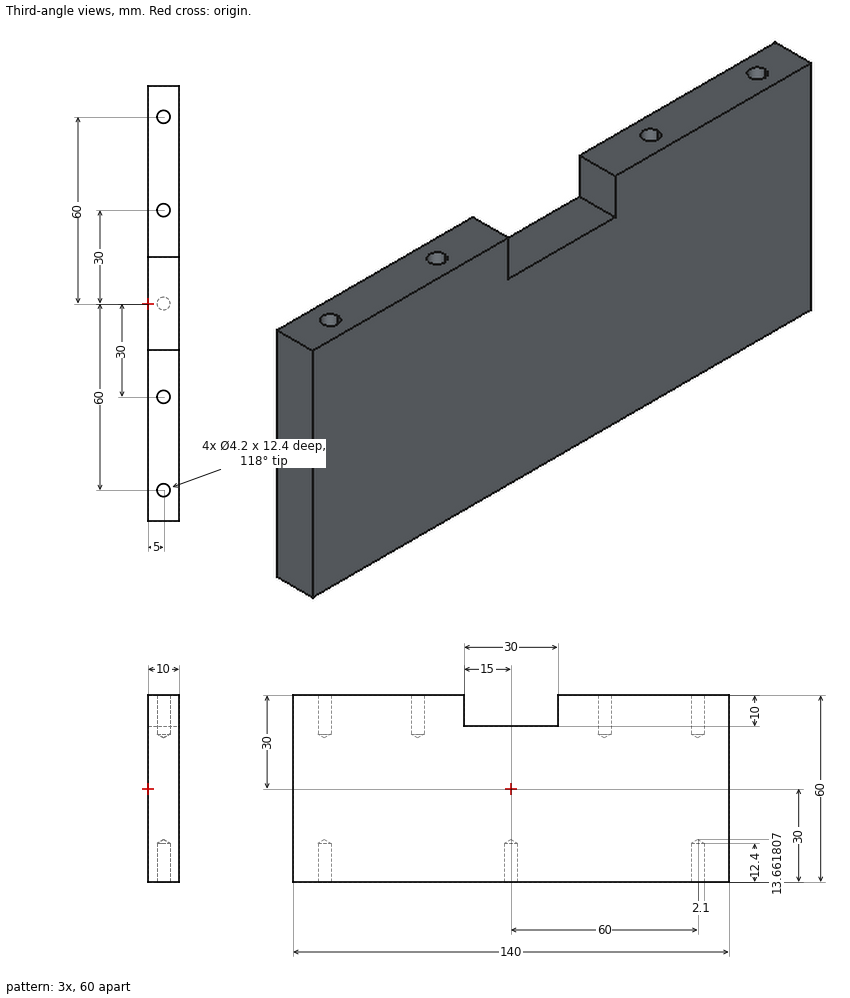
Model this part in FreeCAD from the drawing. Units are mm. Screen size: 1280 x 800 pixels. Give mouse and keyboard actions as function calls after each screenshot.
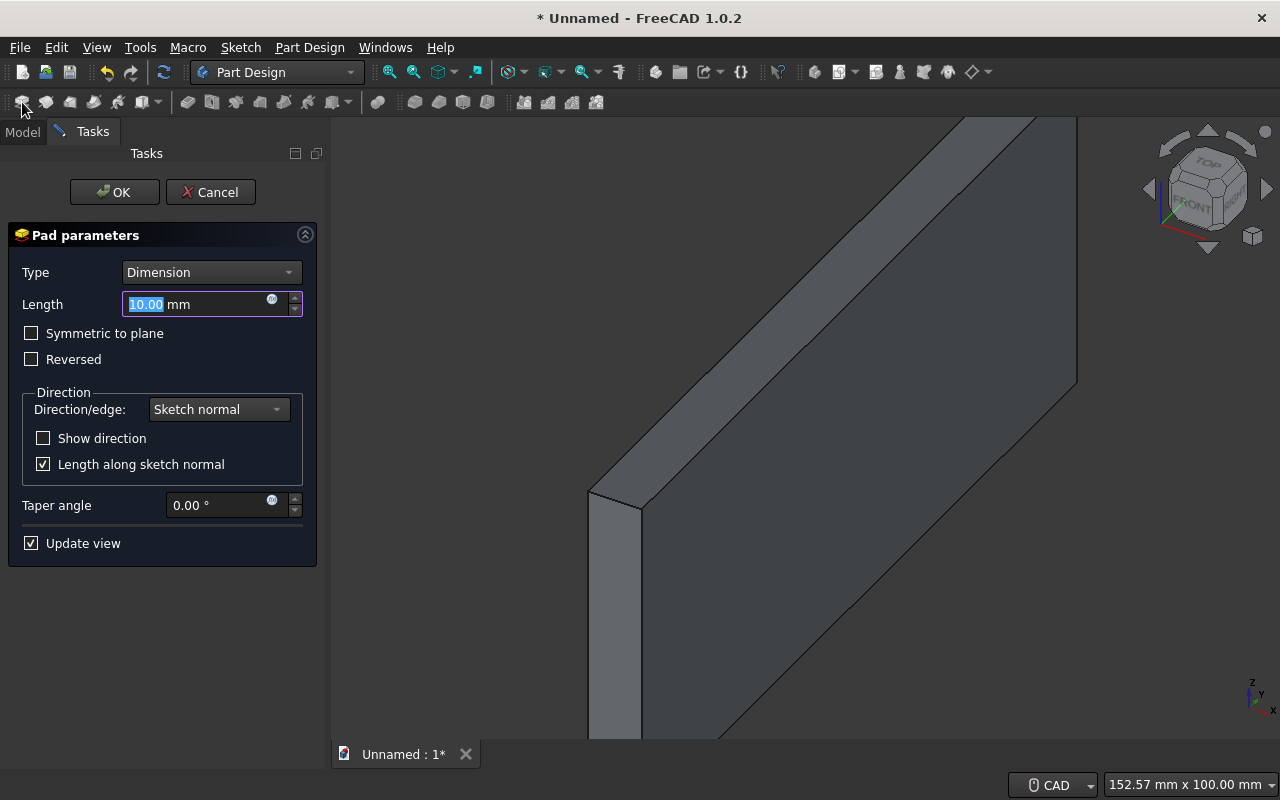
text(10)
key(Tab)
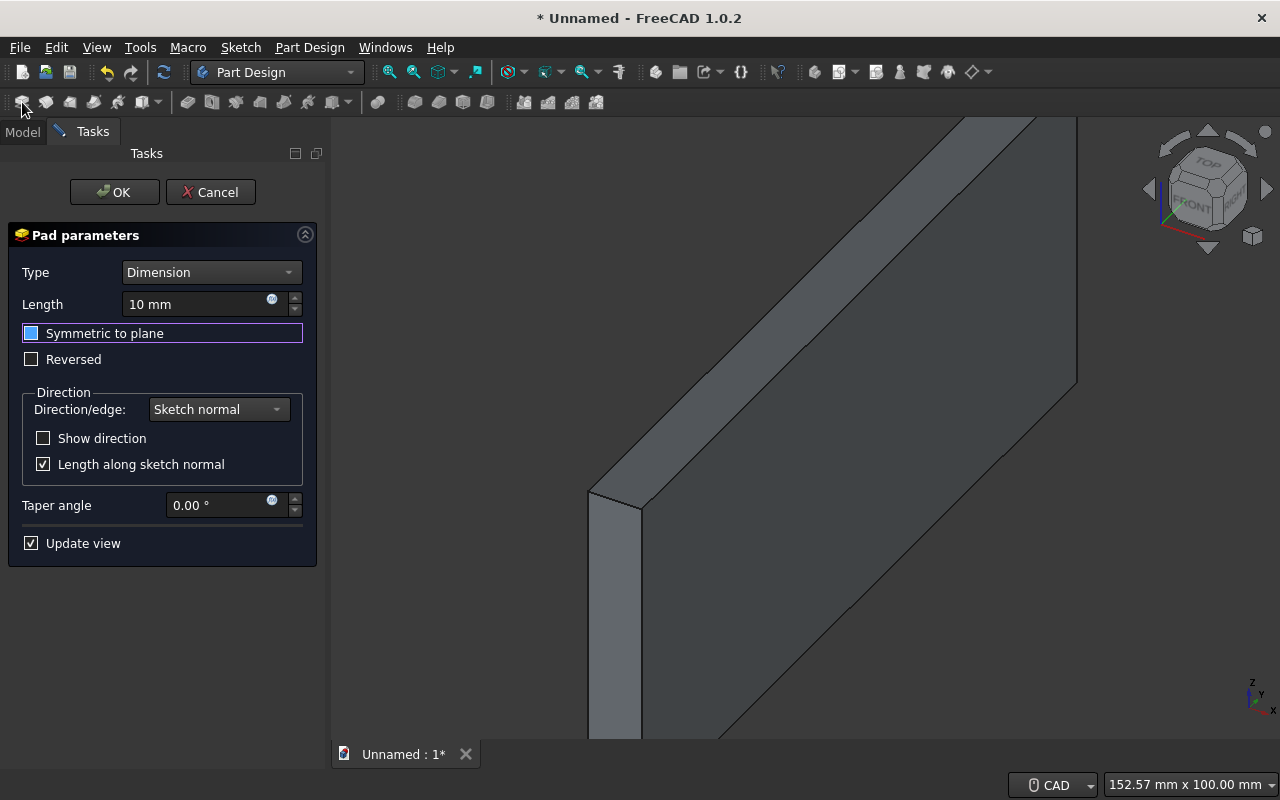
click(115, 192)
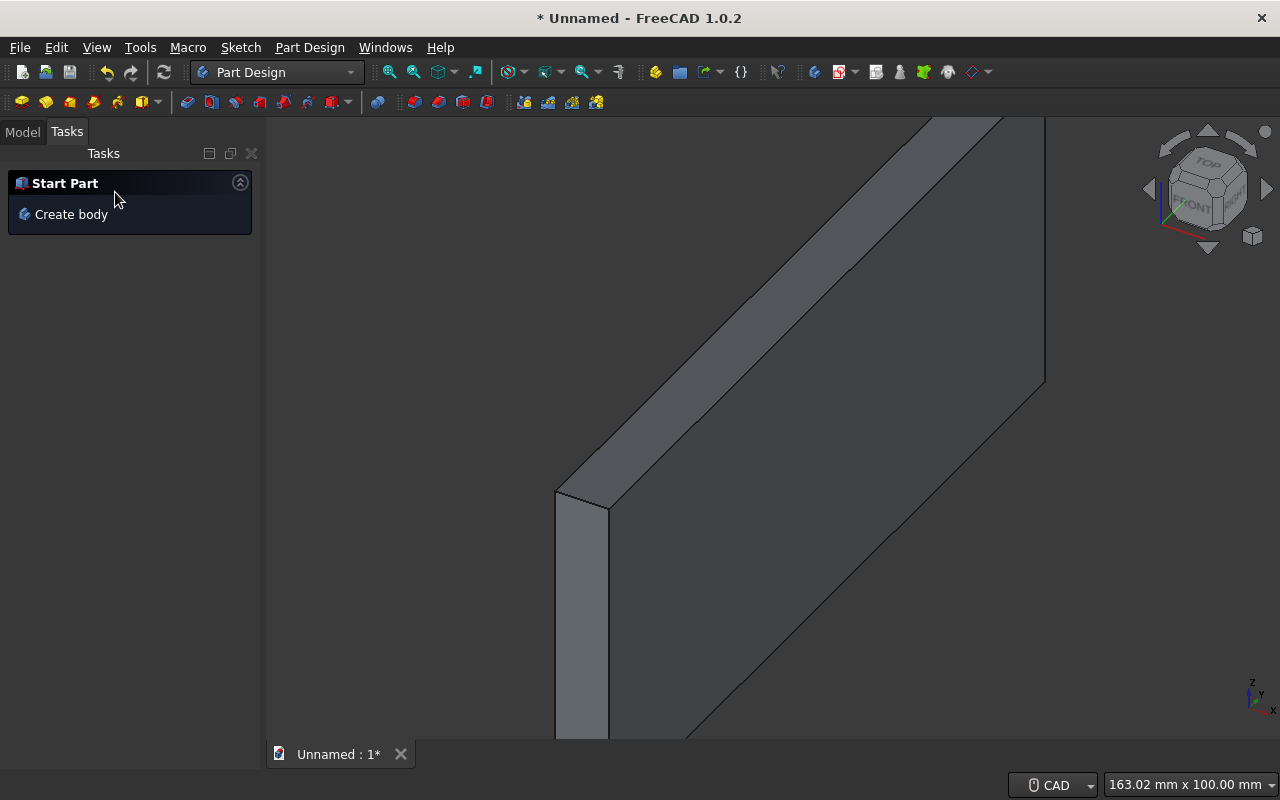
click(390, 72)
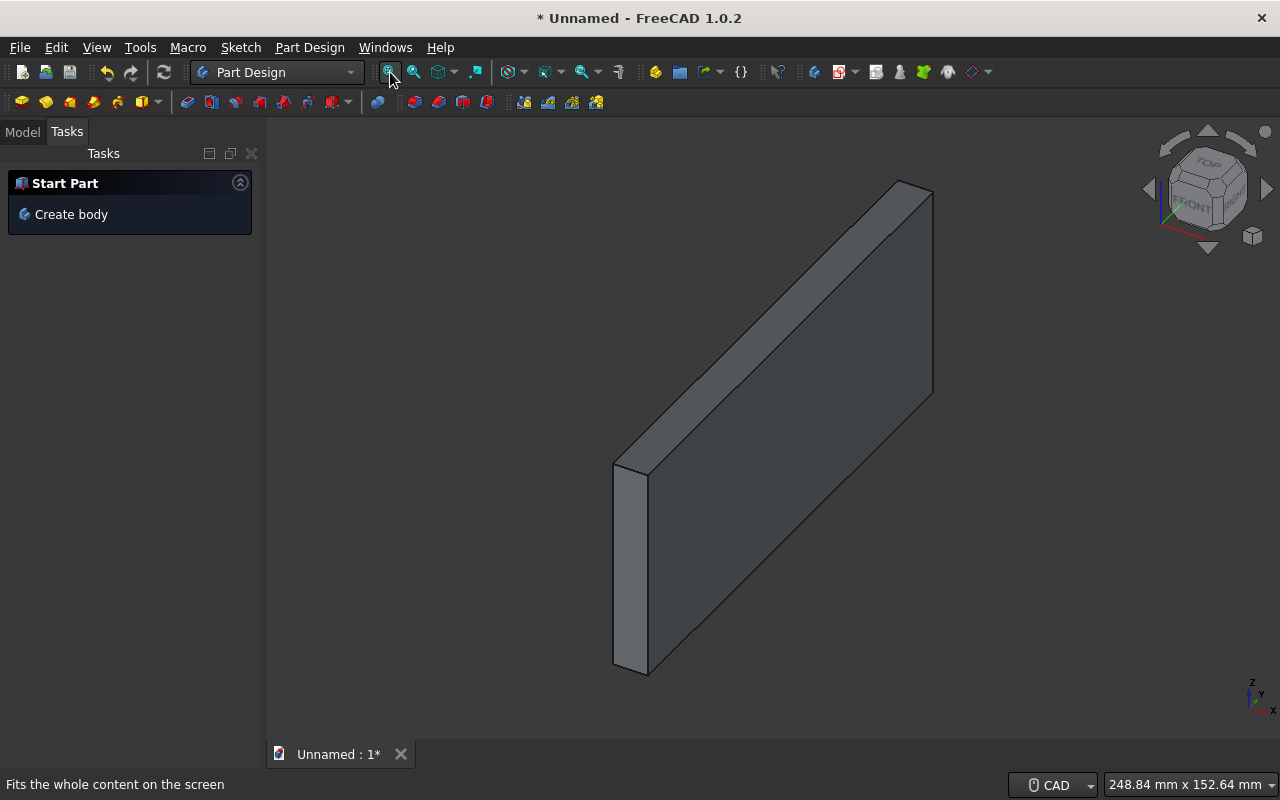
click(840, 72)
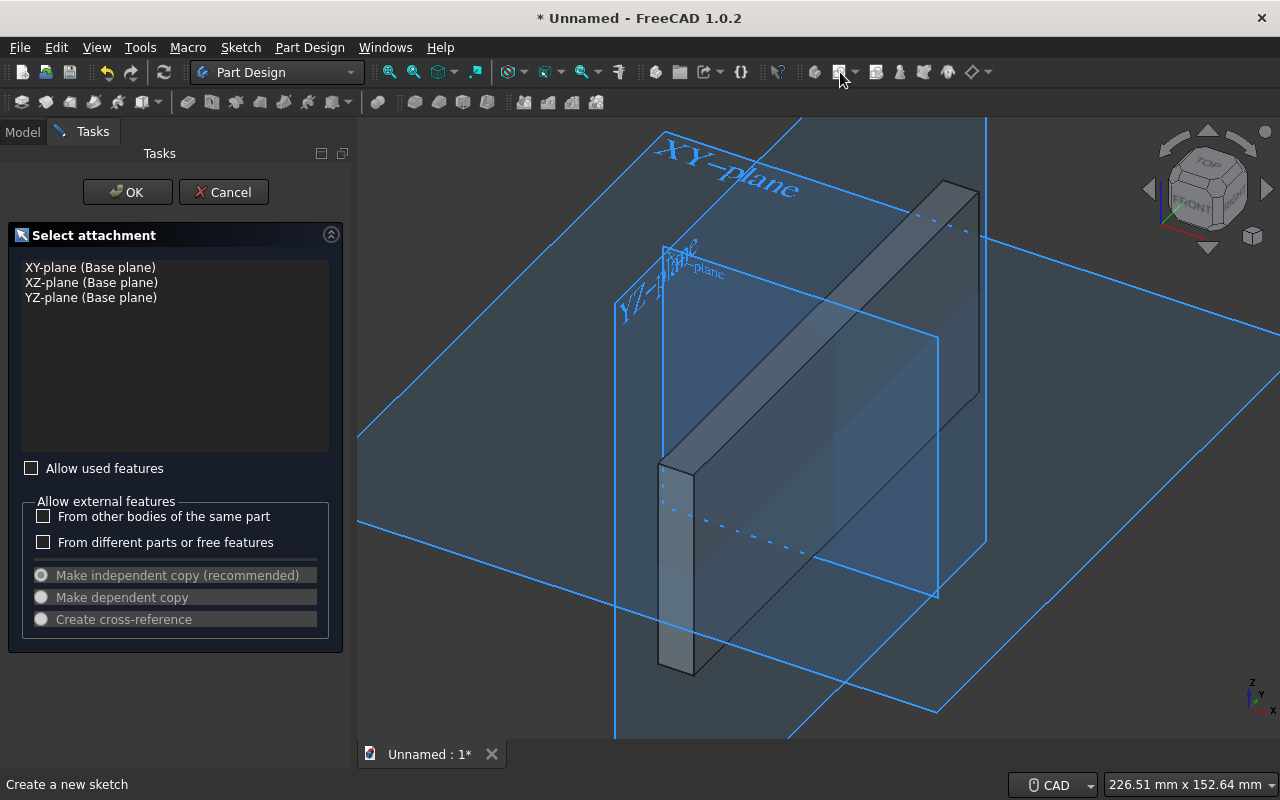
click(82, 298)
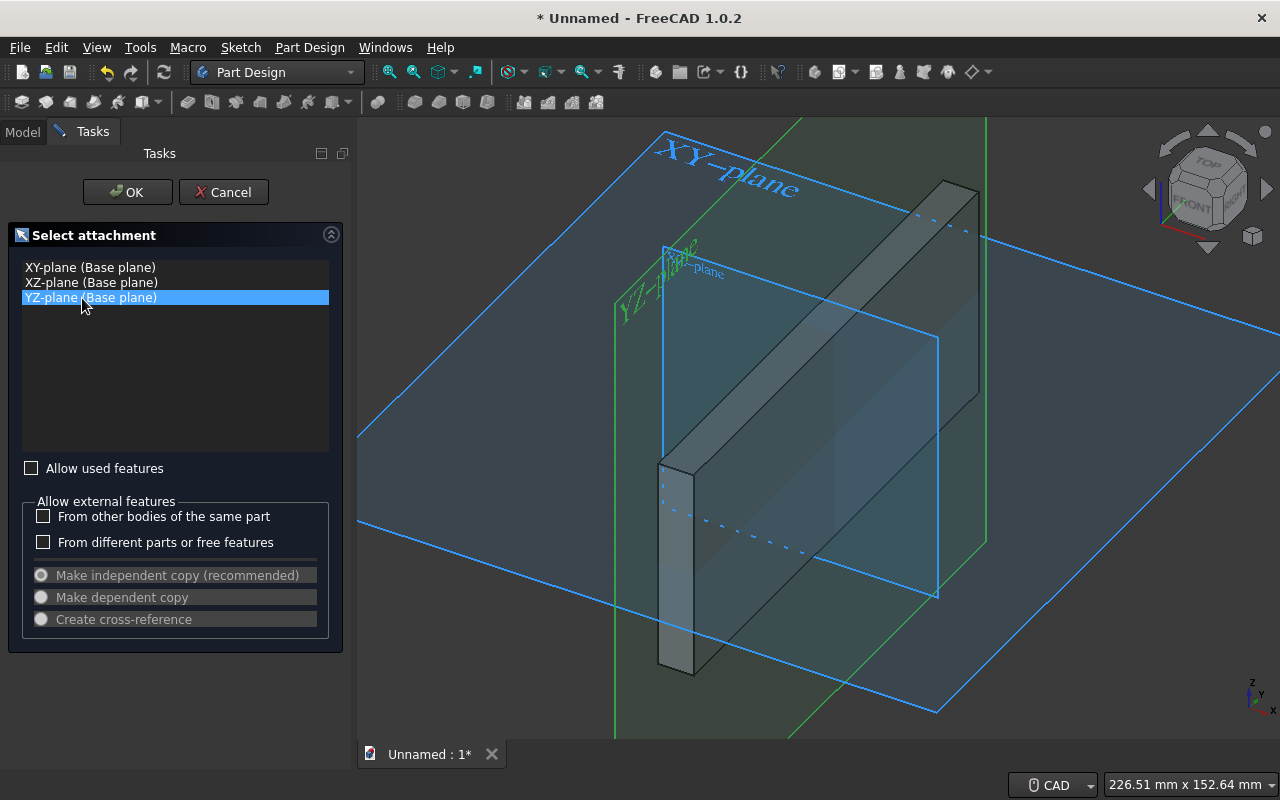
click(128, 192)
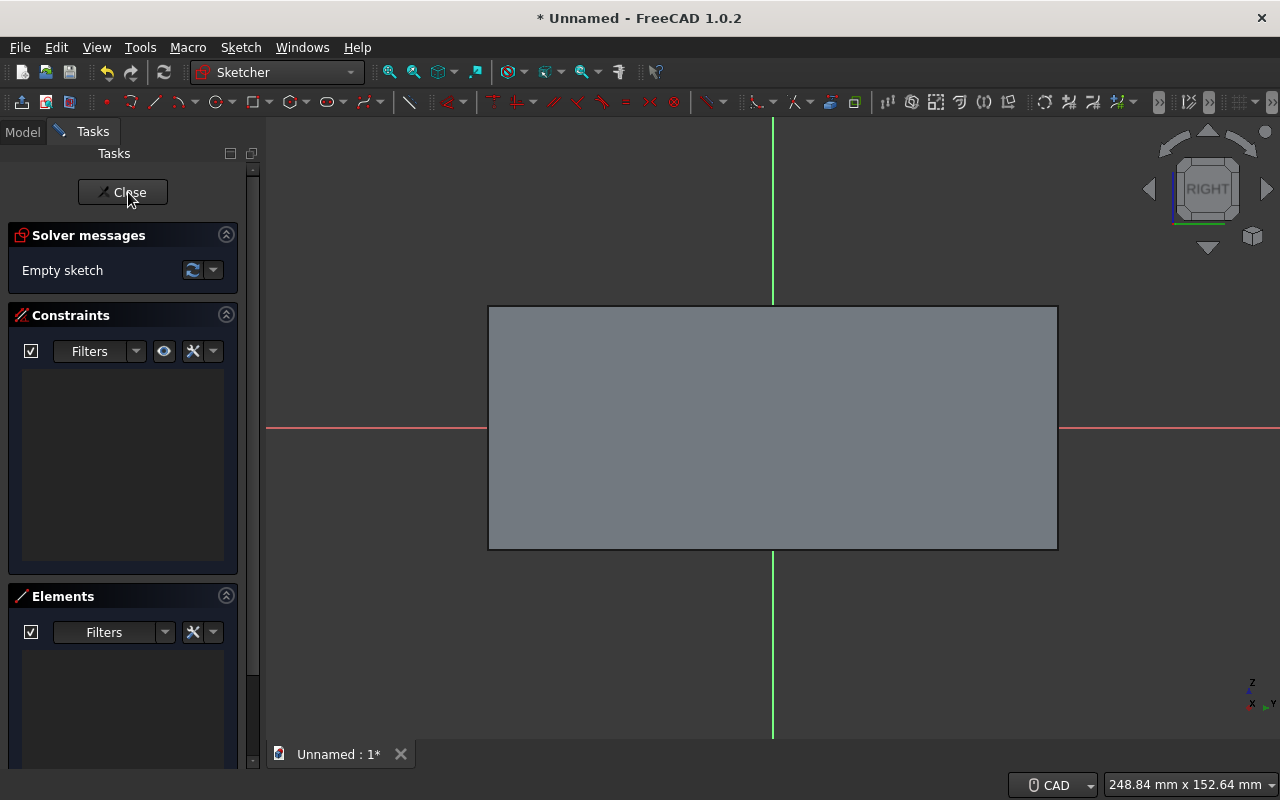
key(q)
key(s)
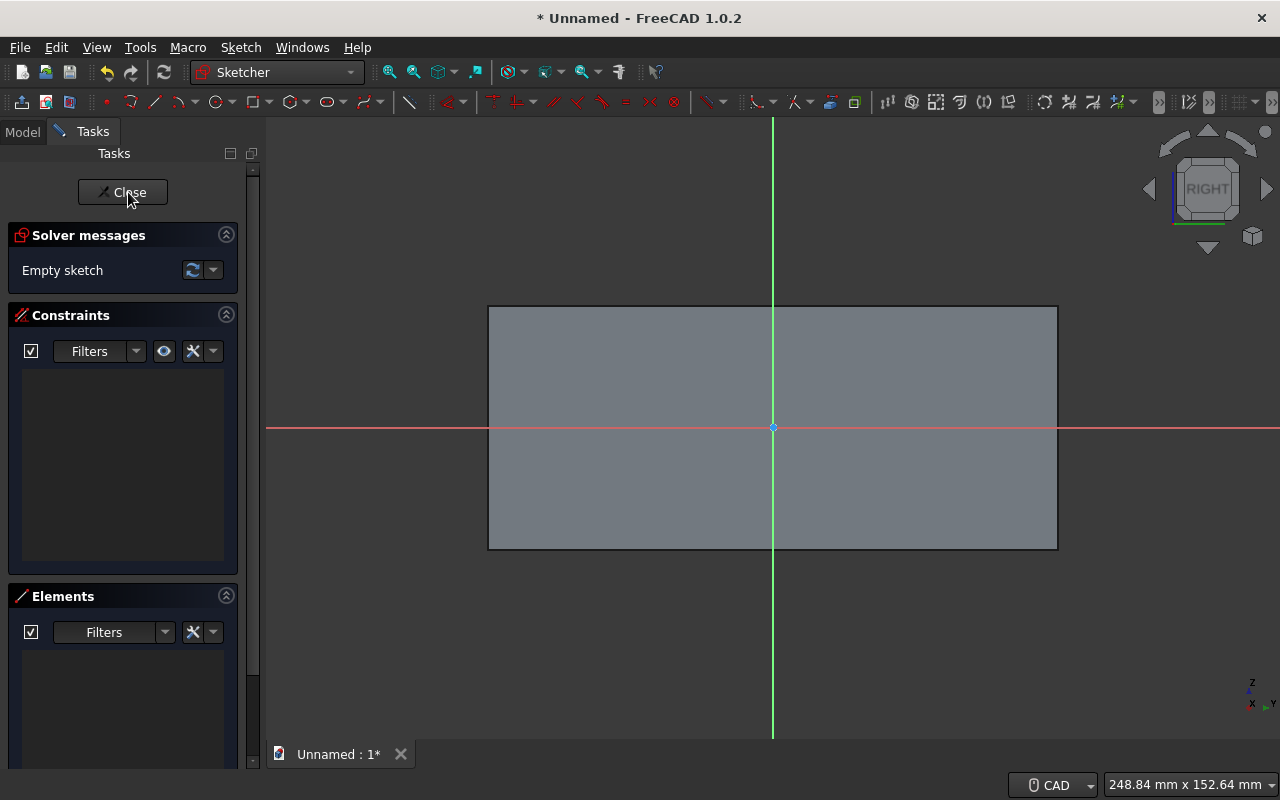
scroll(803, 341, up, 6)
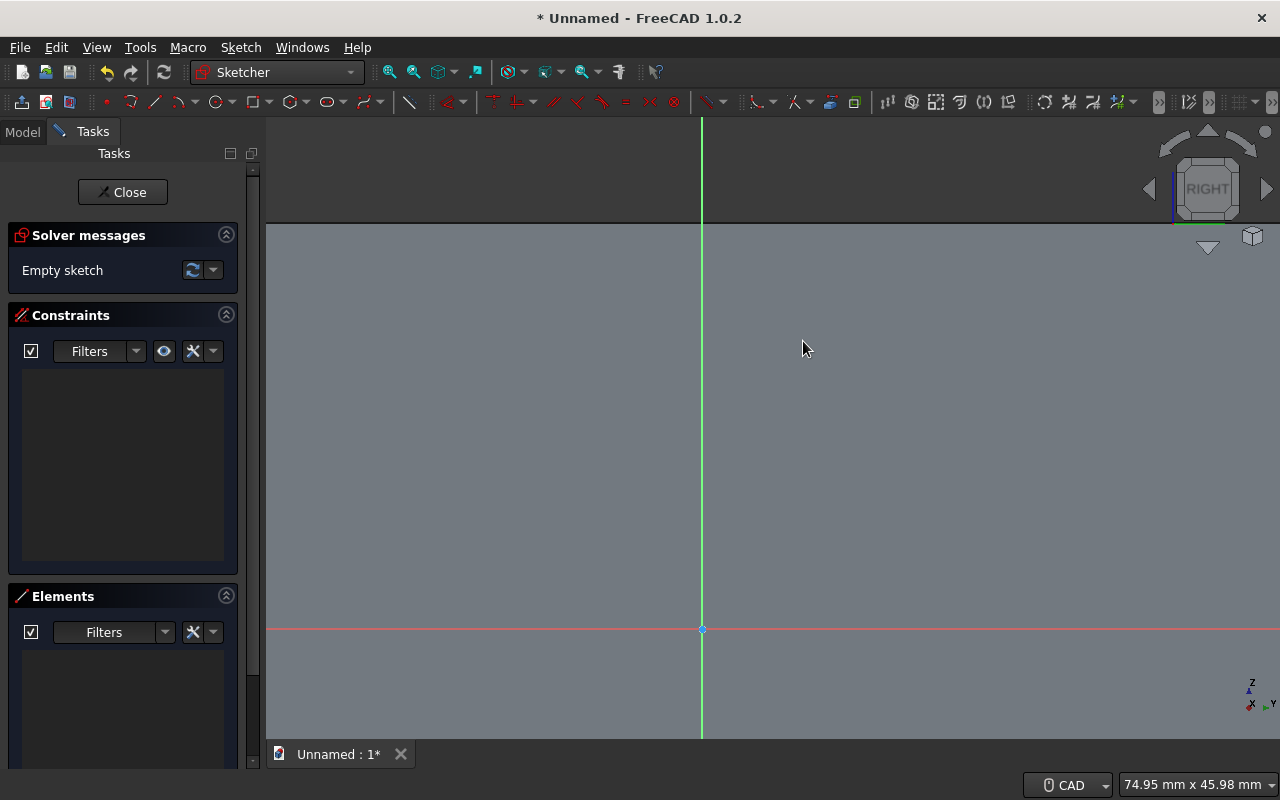
key(g)
key(r)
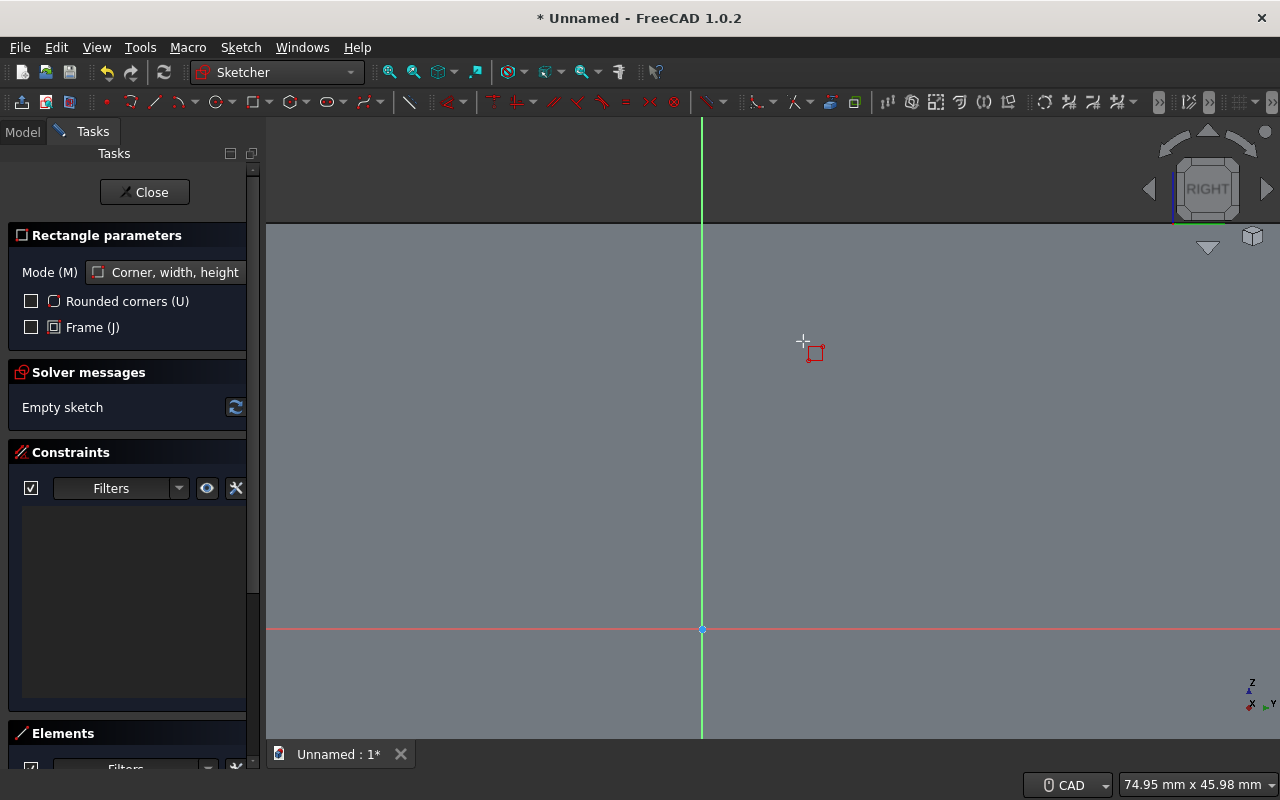
click(499, 223)
move(905, 358)